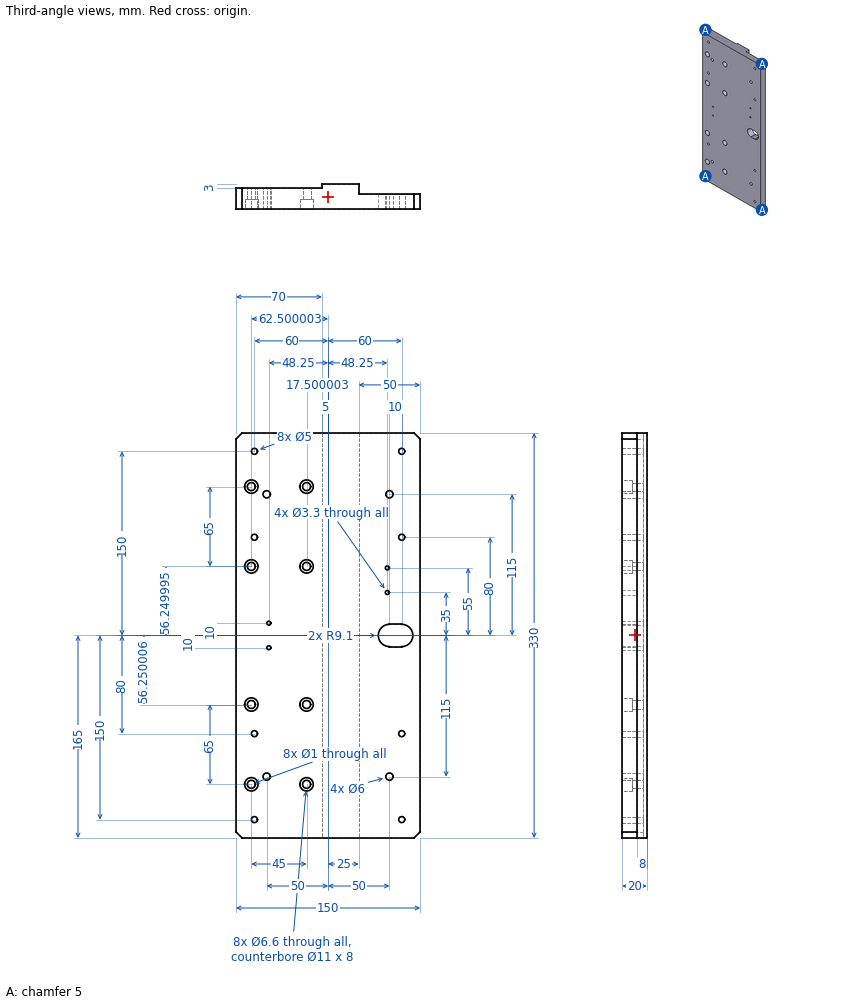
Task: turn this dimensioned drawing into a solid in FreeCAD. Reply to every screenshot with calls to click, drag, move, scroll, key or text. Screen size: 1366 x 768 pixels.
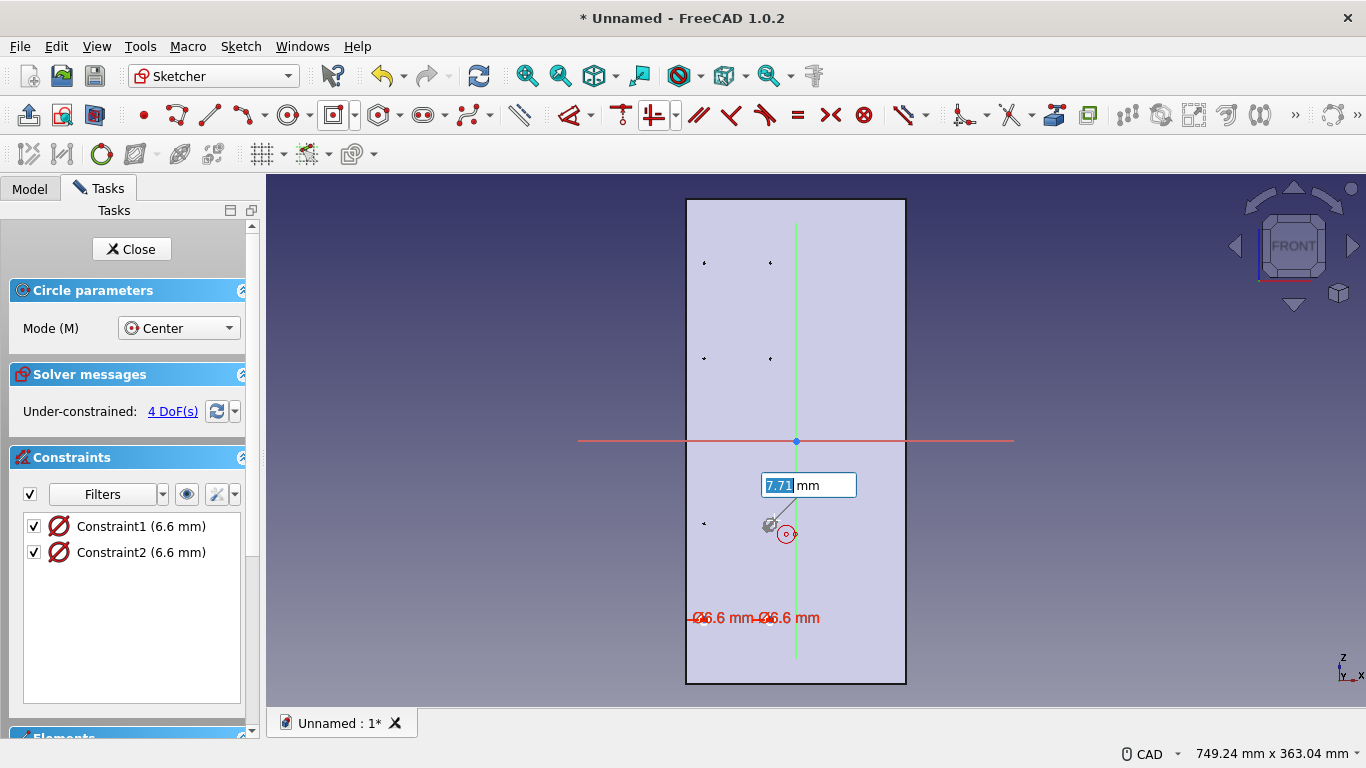
text(6.6)
key(Return)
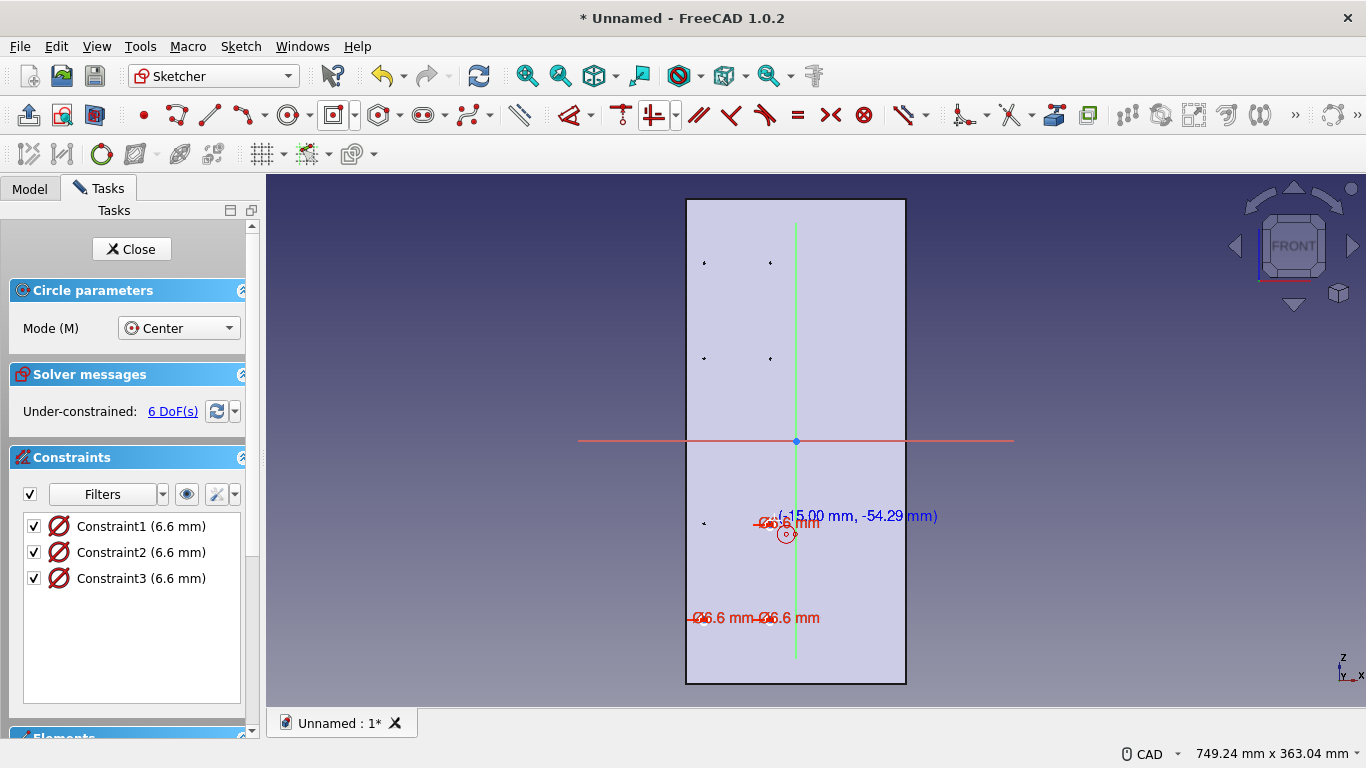
scroll(704, 524, up, 8)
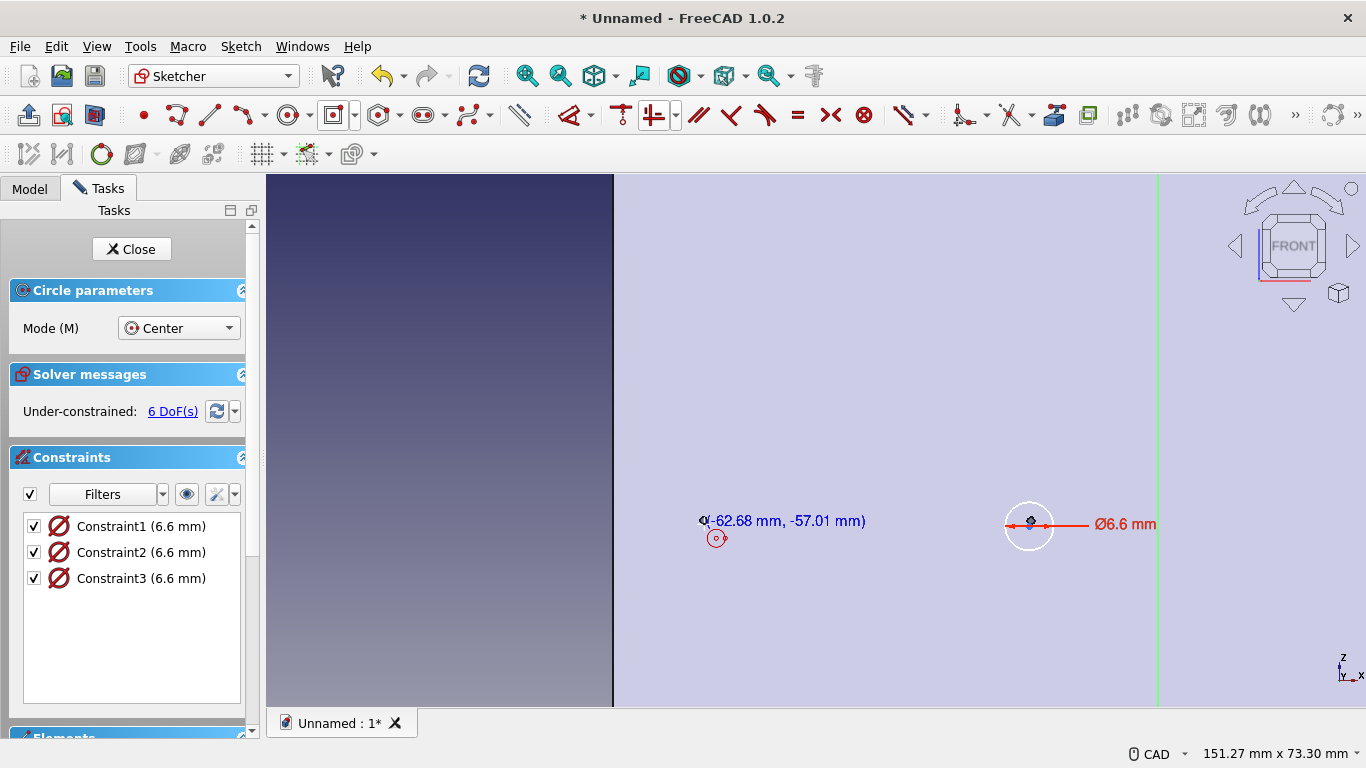
scroll(704, 524, down, 8)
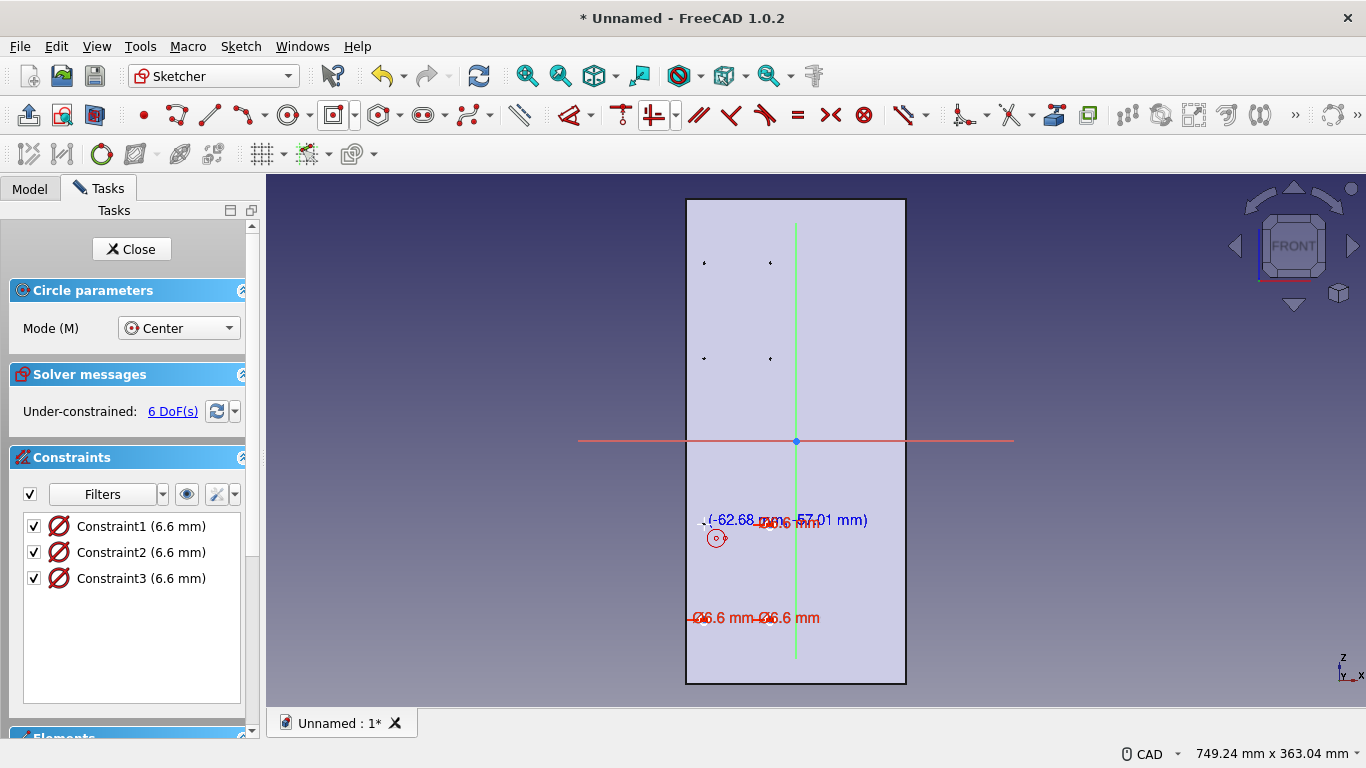
click(704, 524)
move(708, 520)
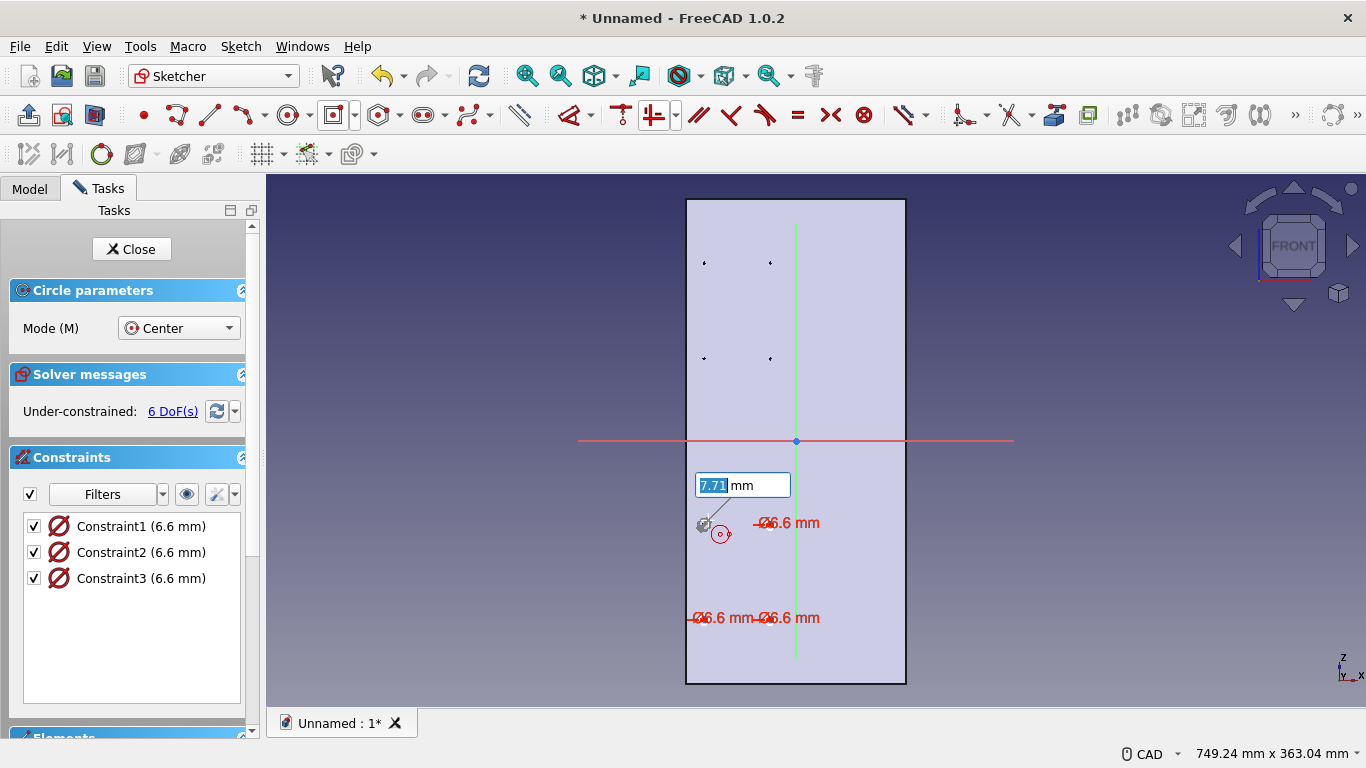
text(6.6)
key(Return)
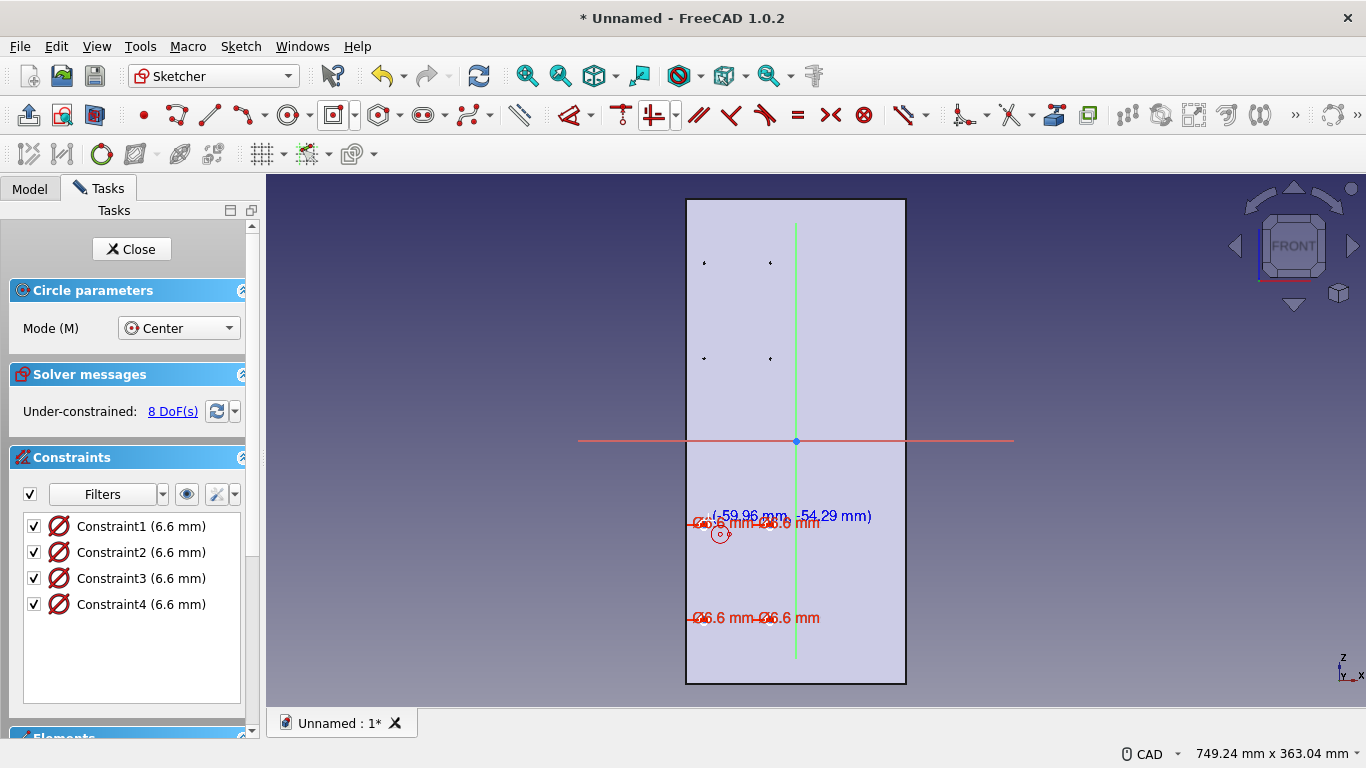
scroll(770, 359, up, 8)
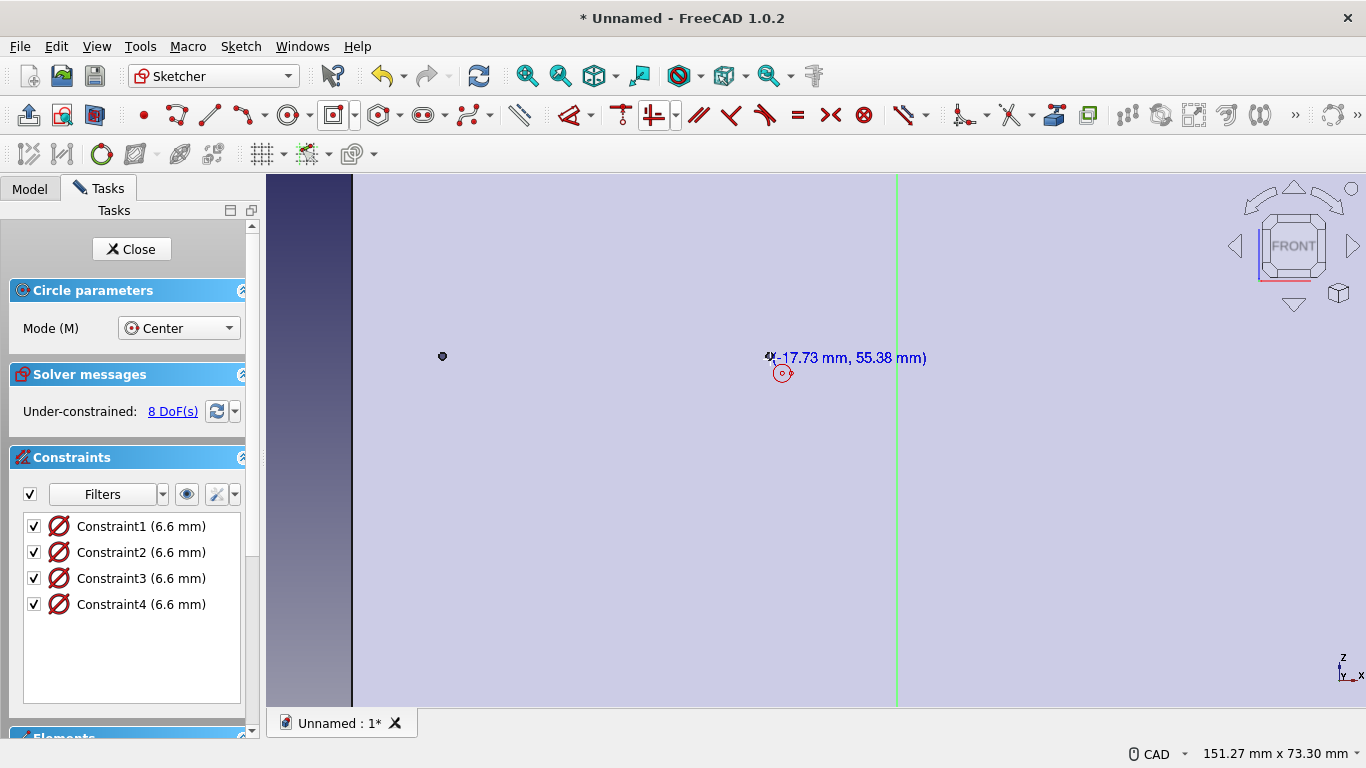
scroll(770, 358, down, 8)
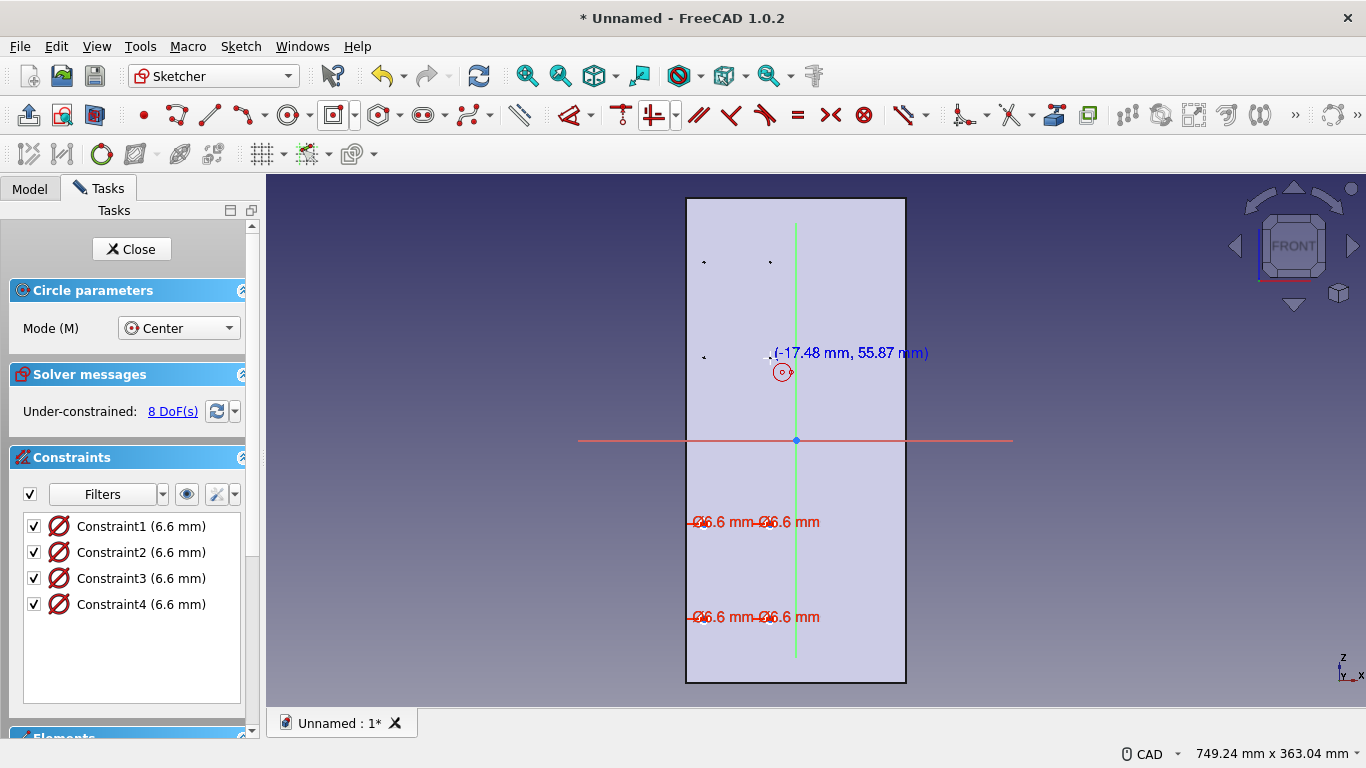
click(770, 358)
move(774, 354)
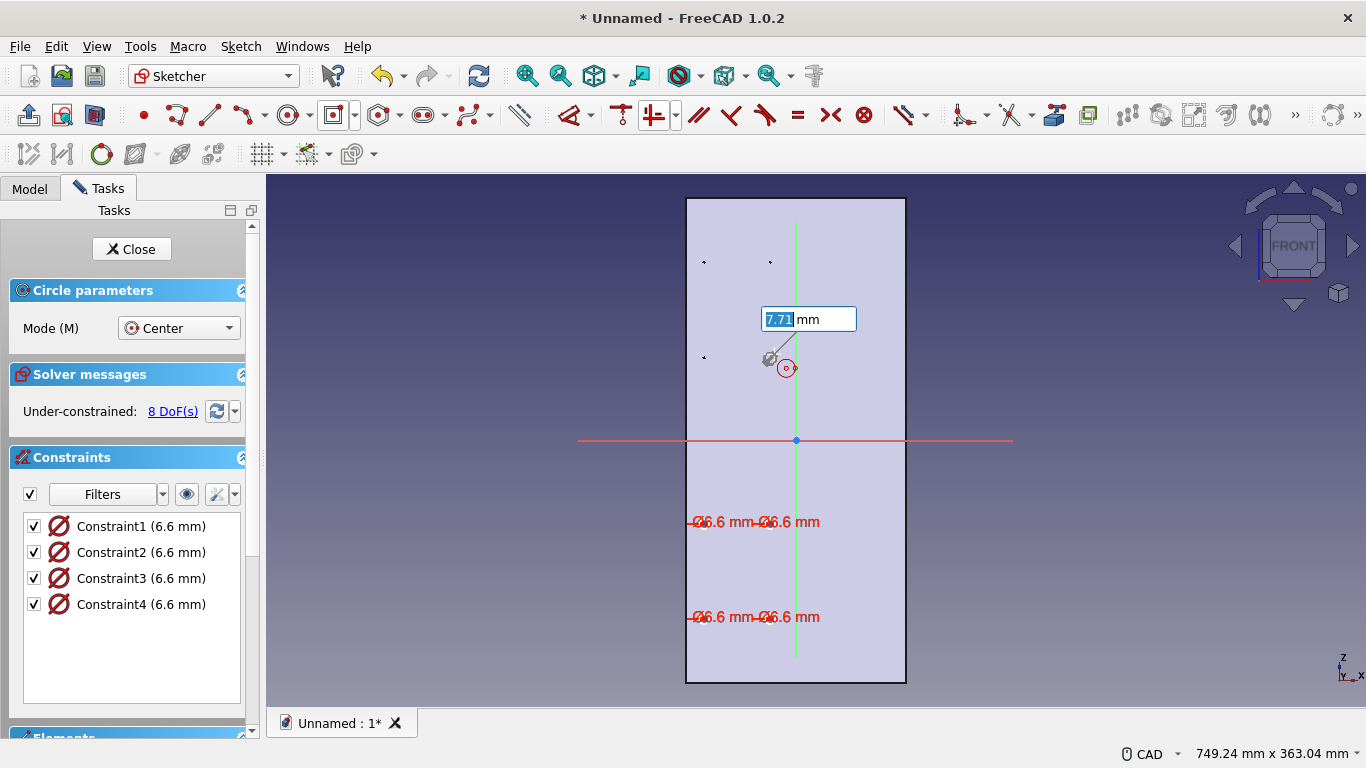
text(6.6)
key(Return)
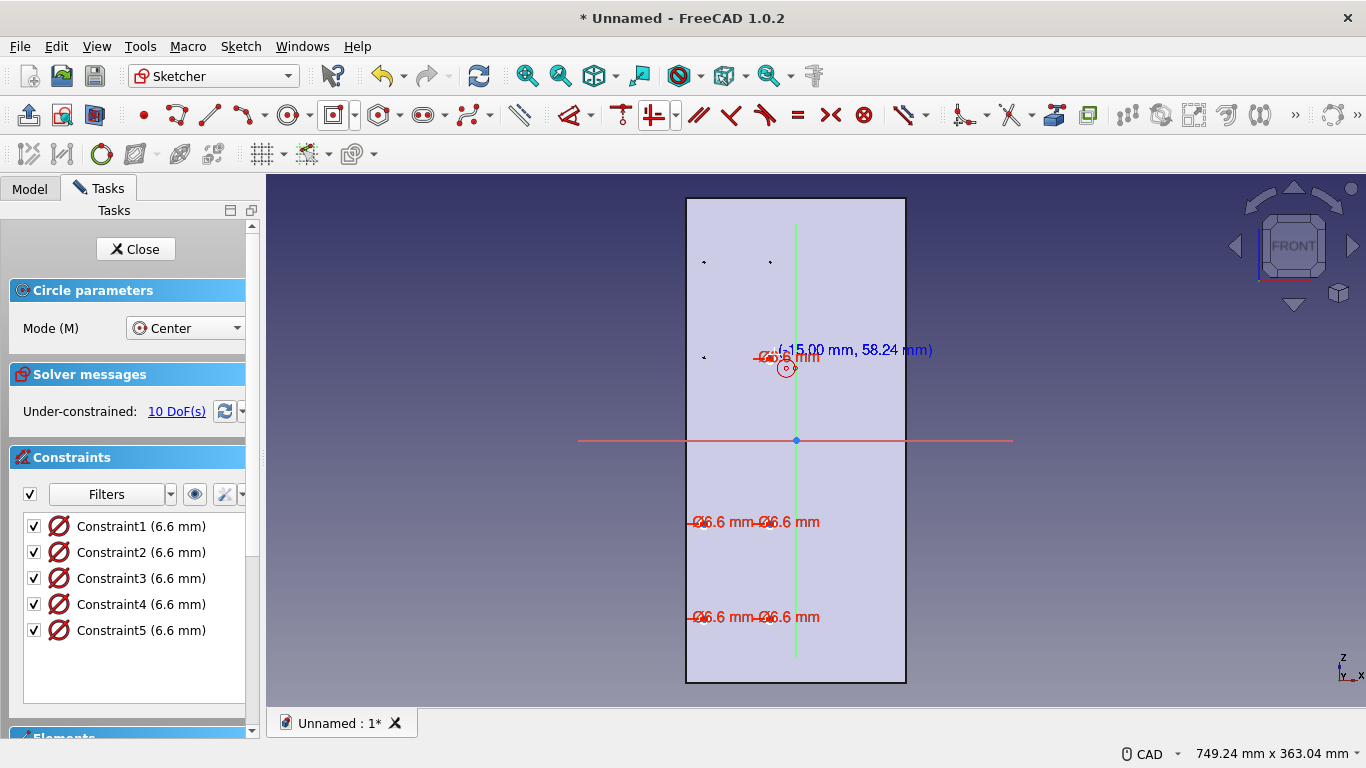
scroll(704, 358, up, 8)